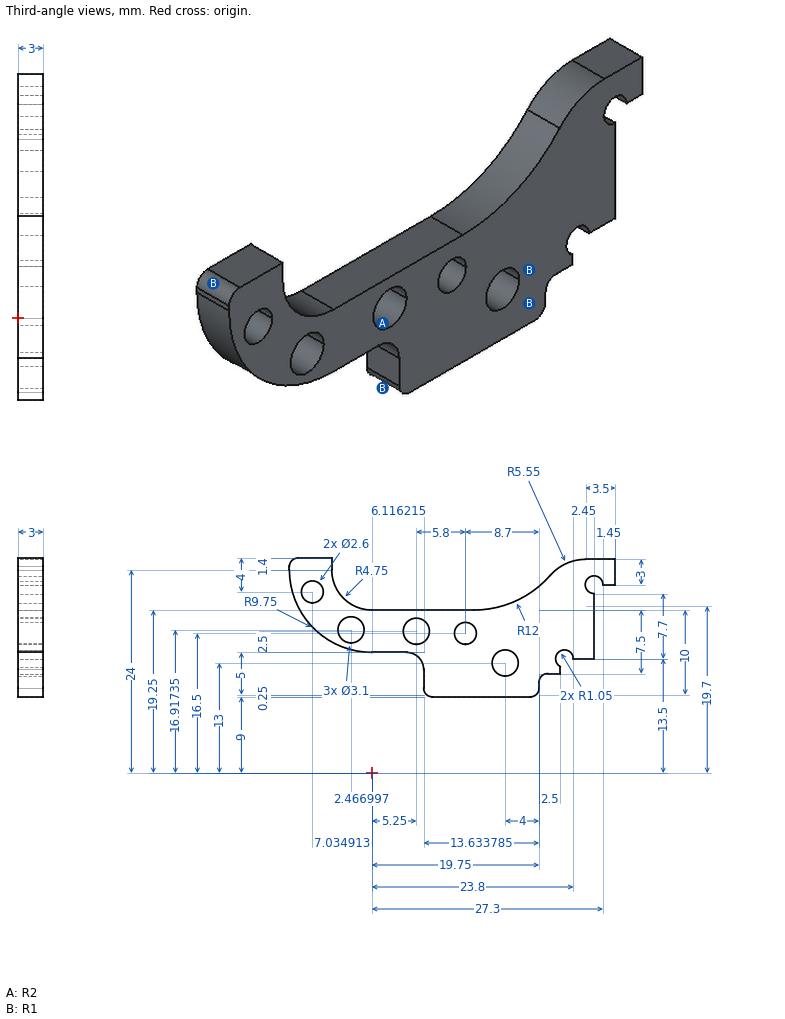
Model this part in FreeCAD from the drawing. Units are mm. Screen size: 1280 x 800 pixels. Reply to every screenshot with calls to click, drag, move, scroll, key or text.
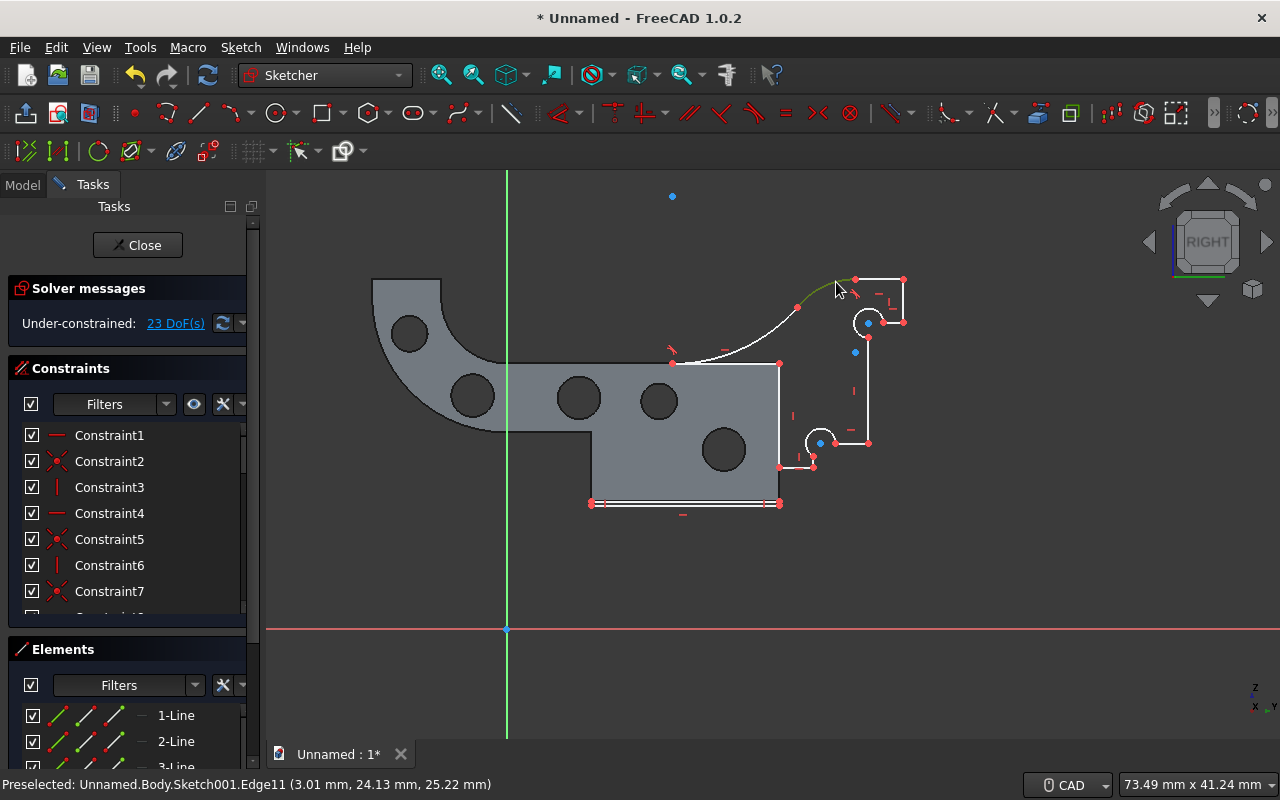
click(766, 335)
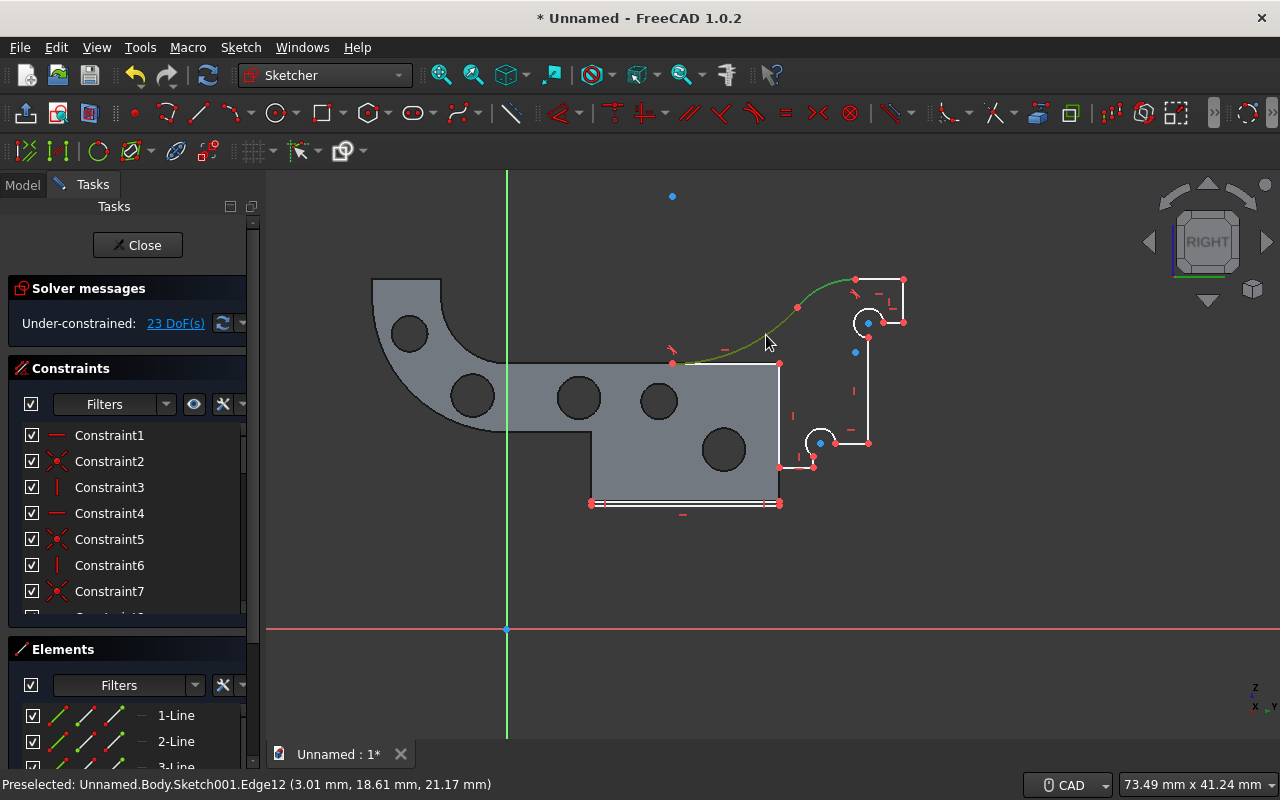
key(t)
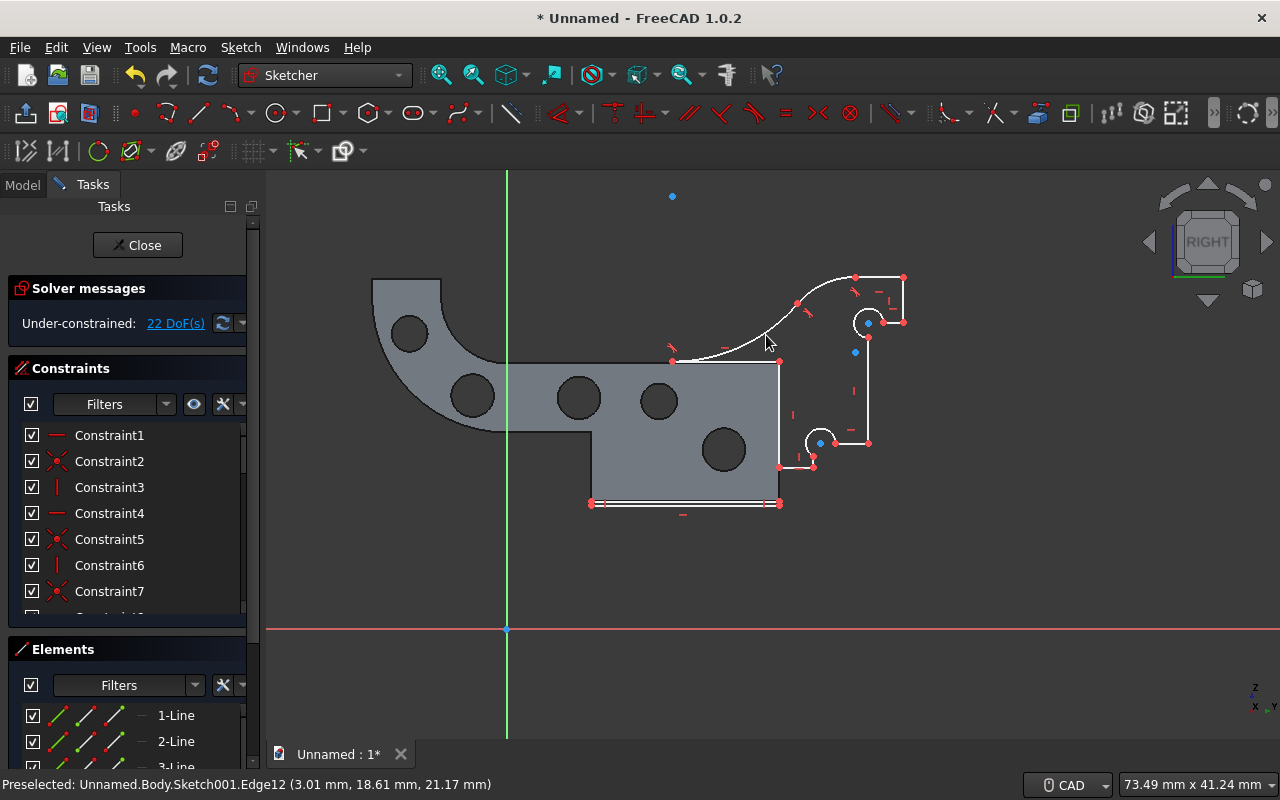
click(871, 309)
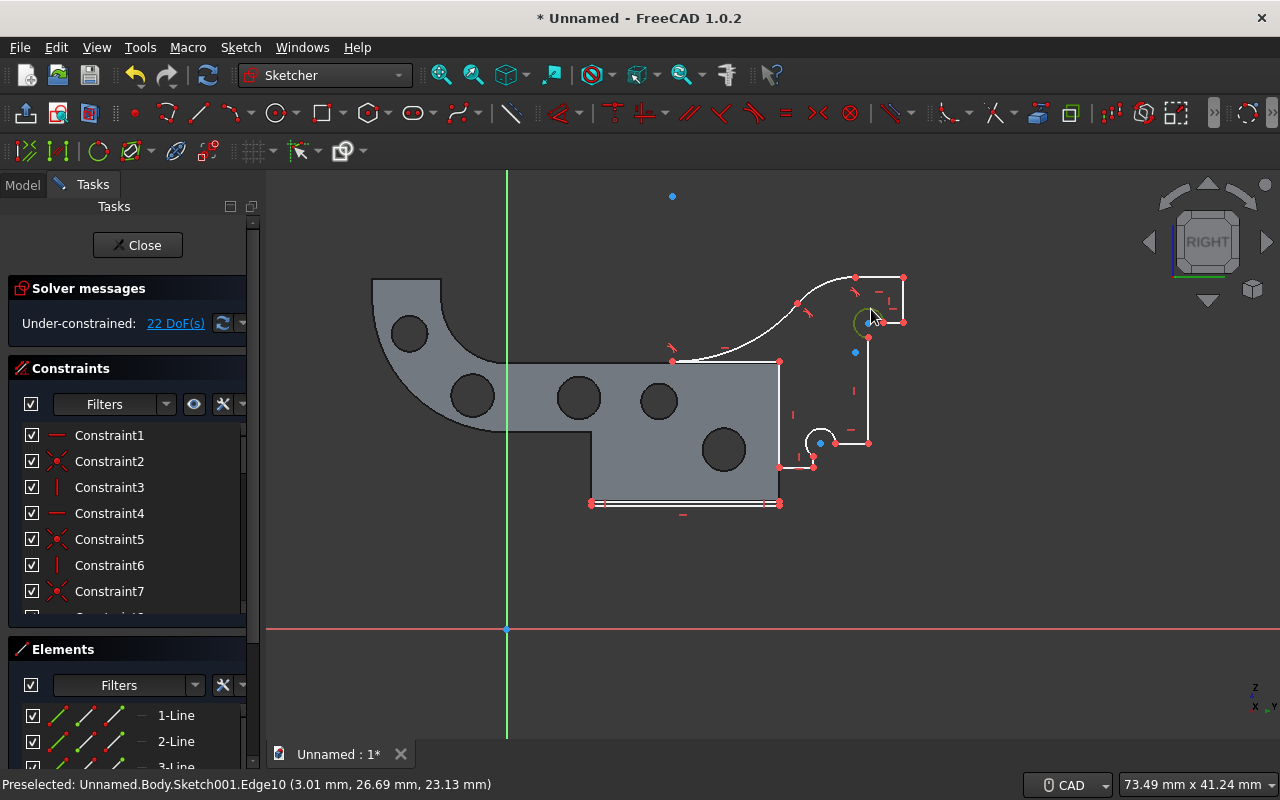
click(826, 429)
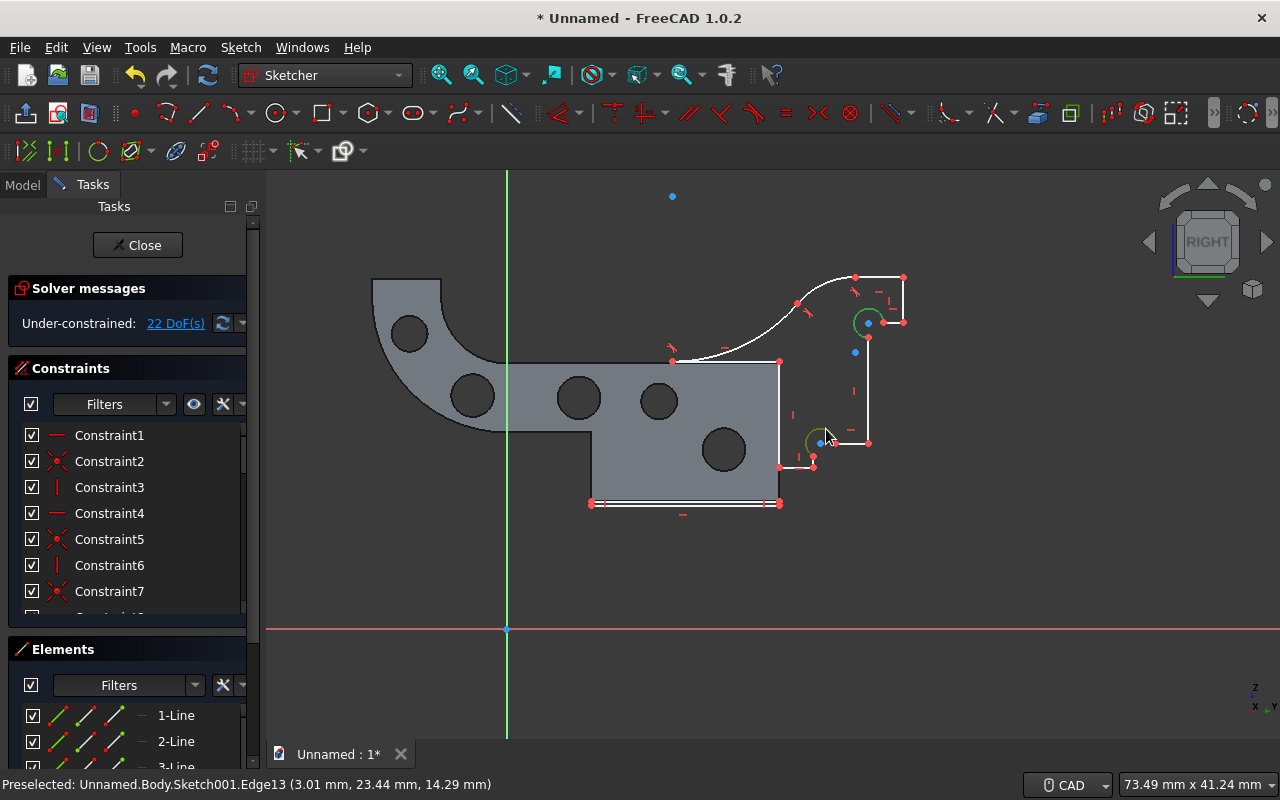
click(786, 114)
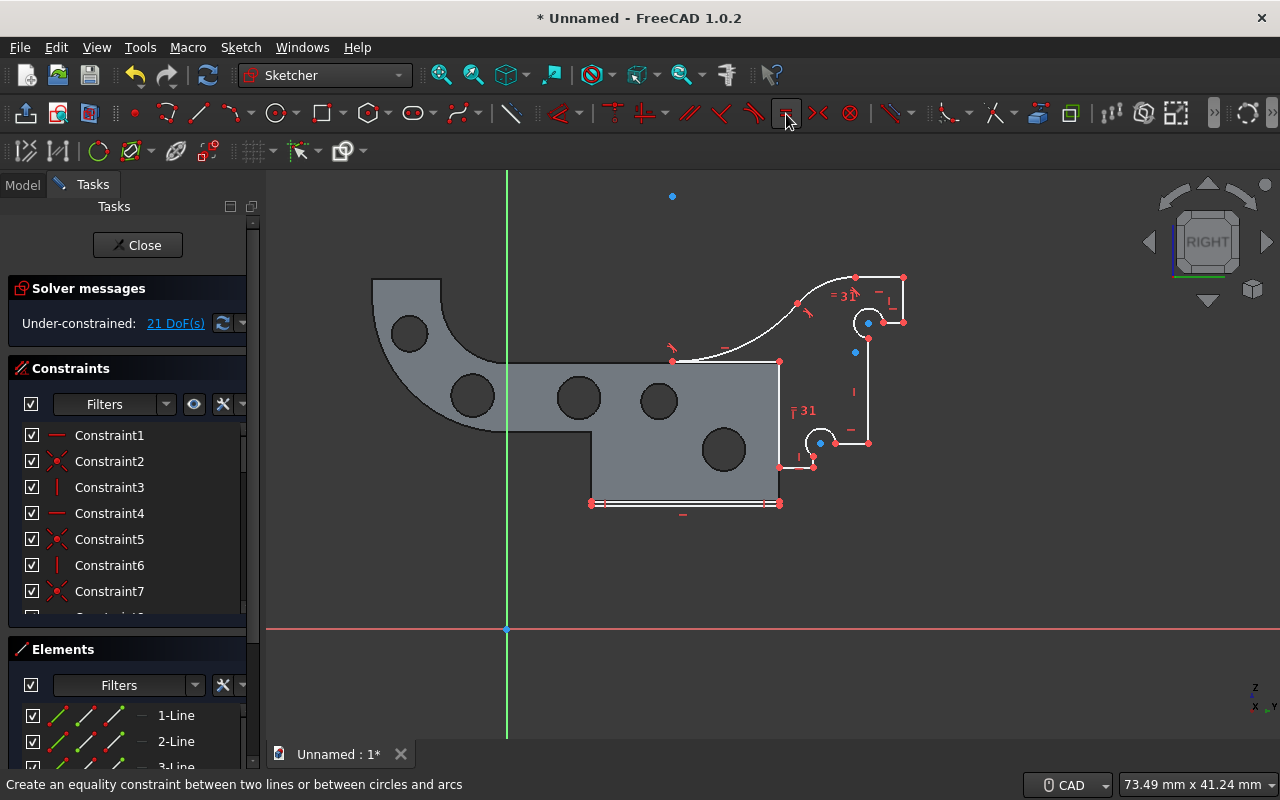
key(d)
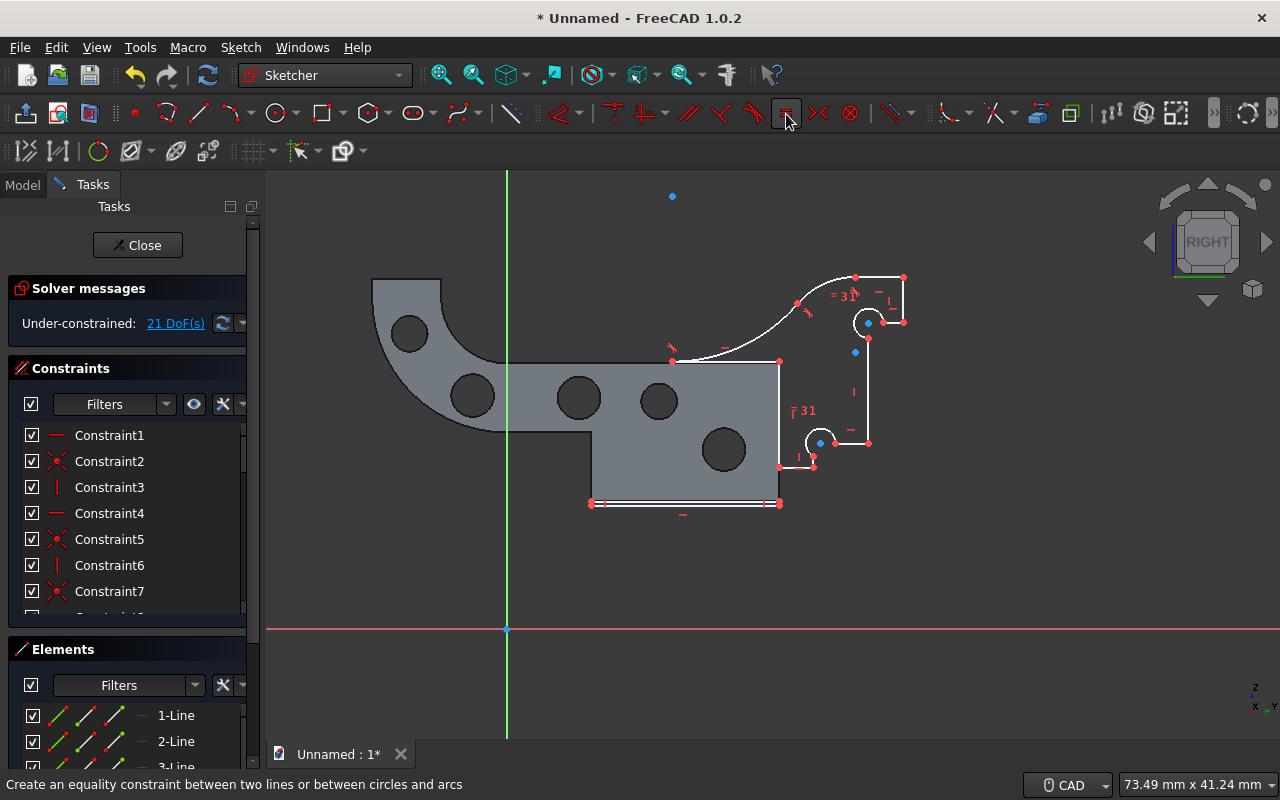
scroll(871, 309, up, 6)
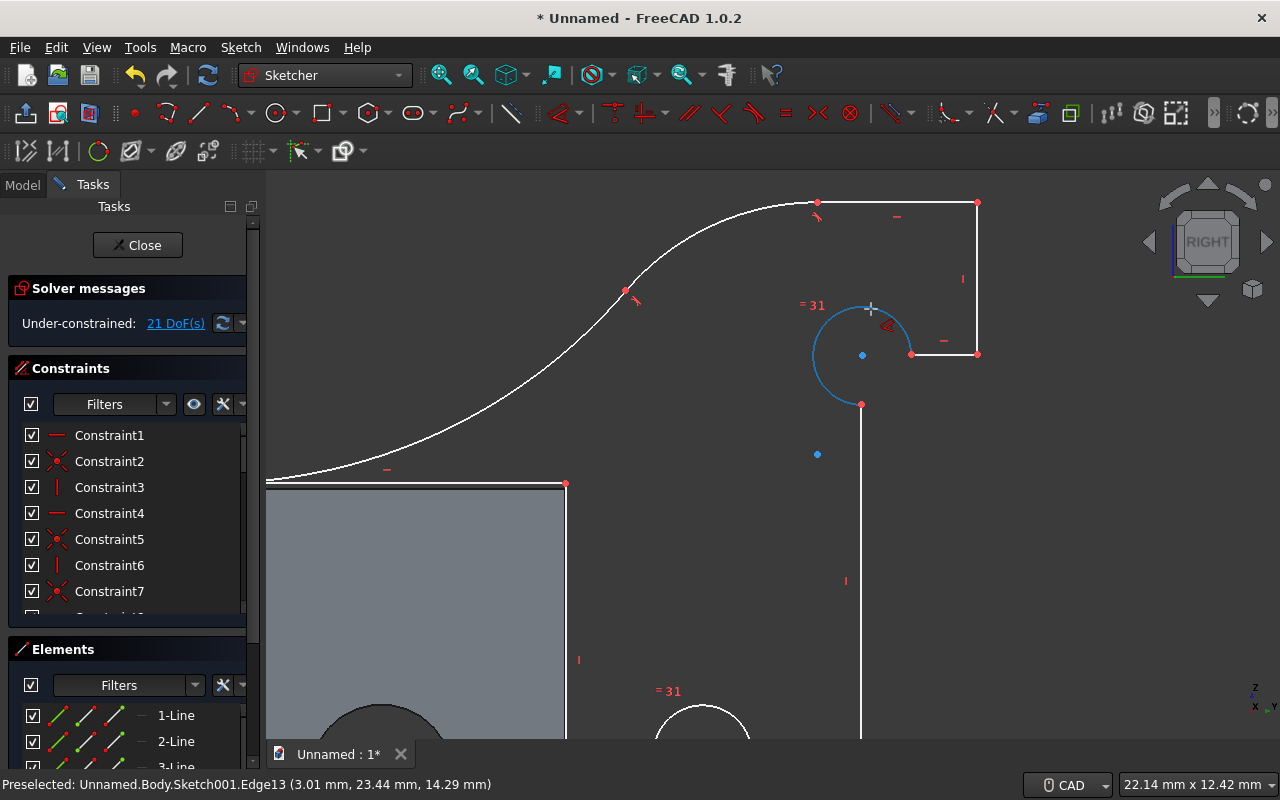
click(869, 307)
click(873, 275)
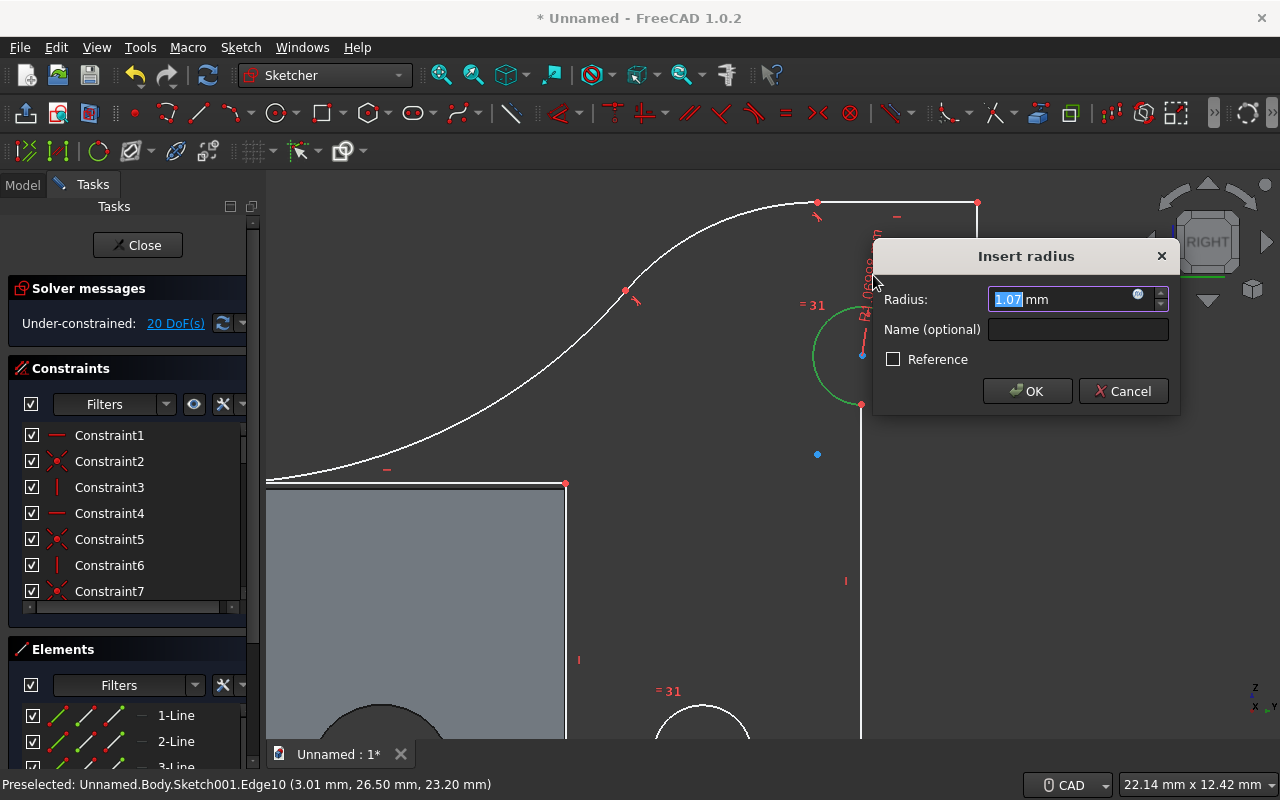
text(1.05)
key(Return)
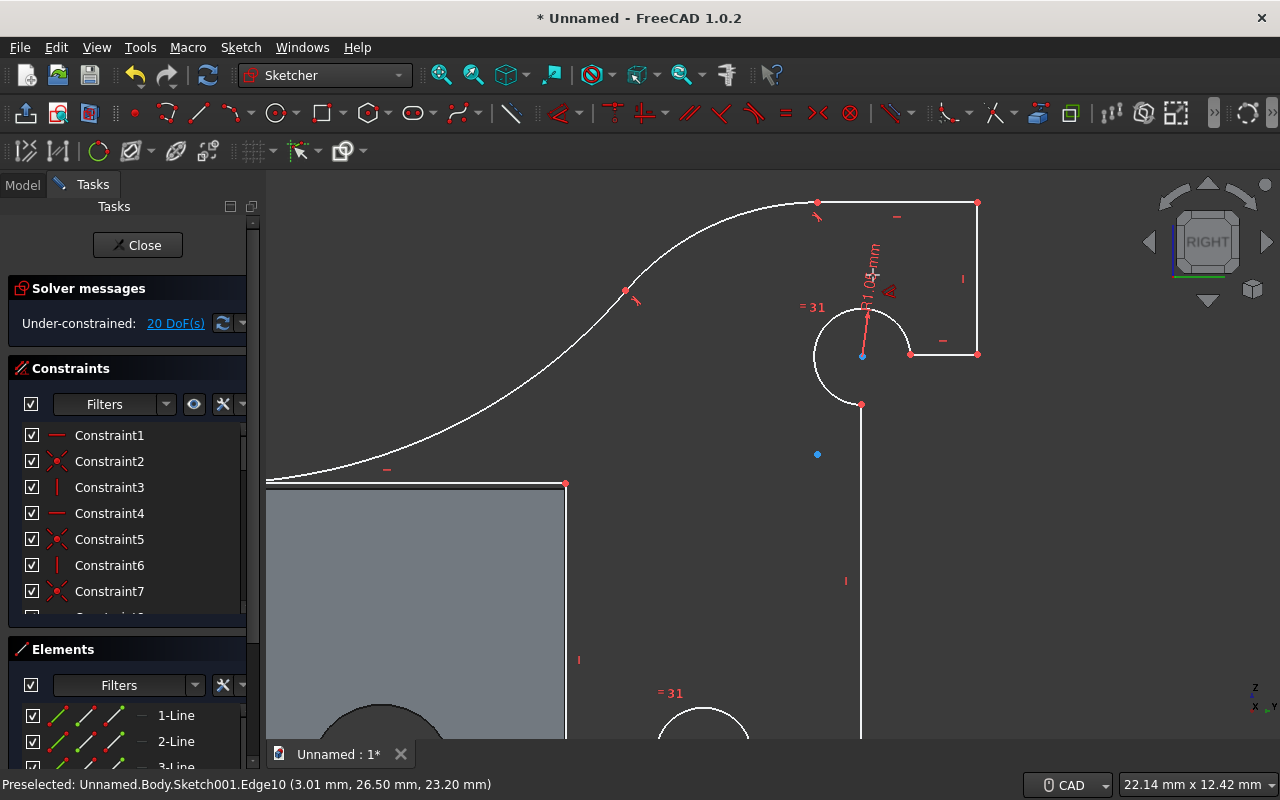
click(753, 211)
click(622, 249)